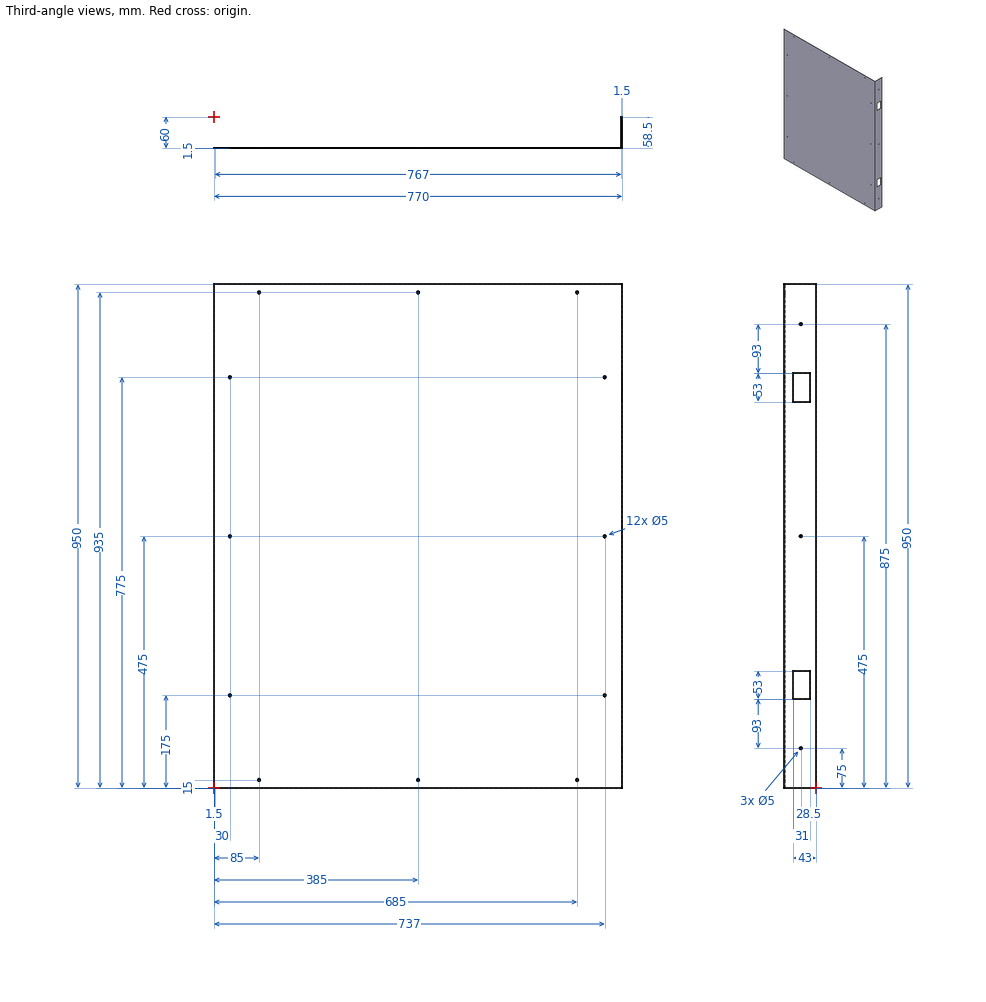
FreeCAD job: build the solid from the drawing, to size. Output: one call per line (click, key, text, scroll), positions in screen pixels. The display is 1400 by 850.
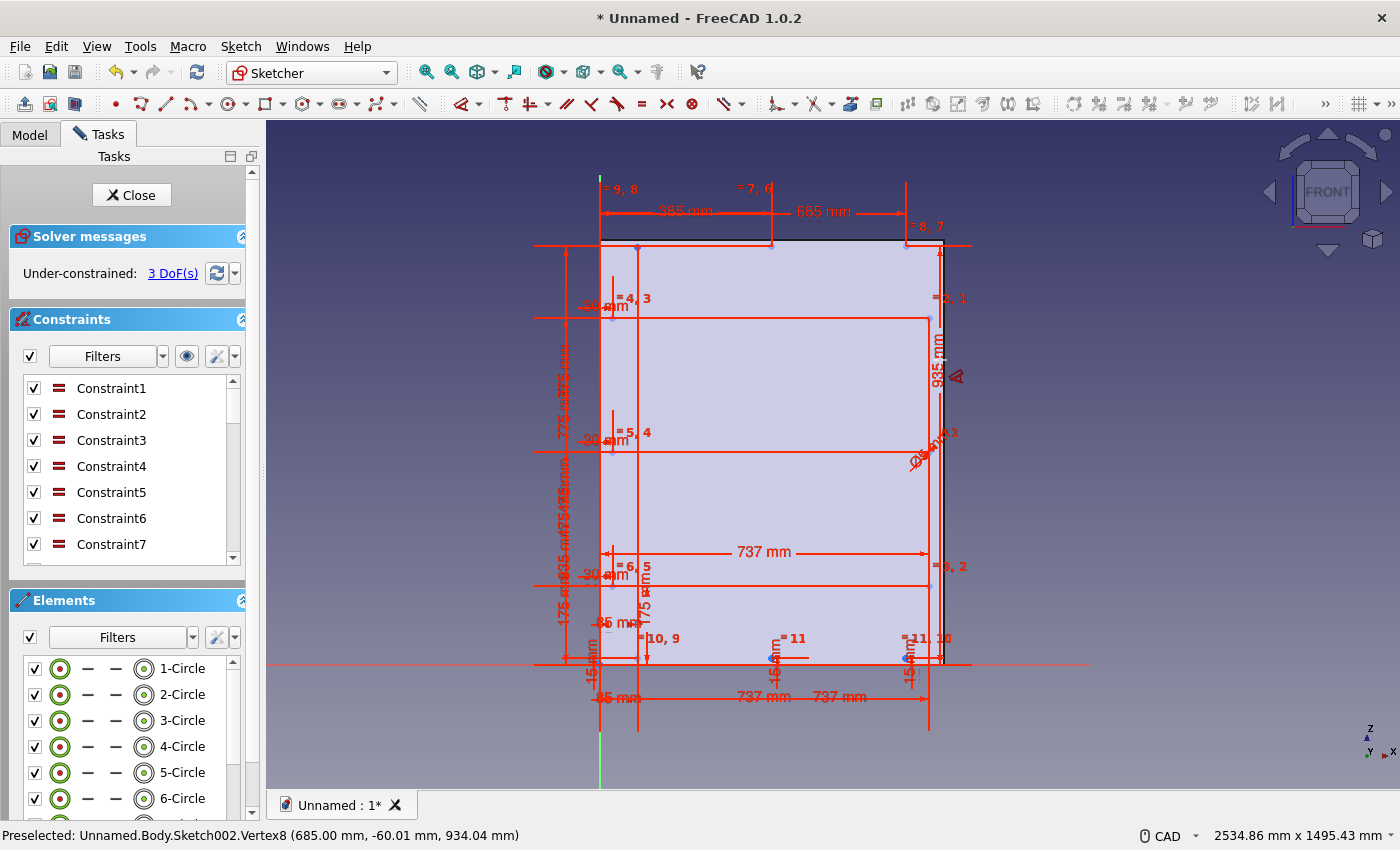
click(638, 247)
click(672, 360)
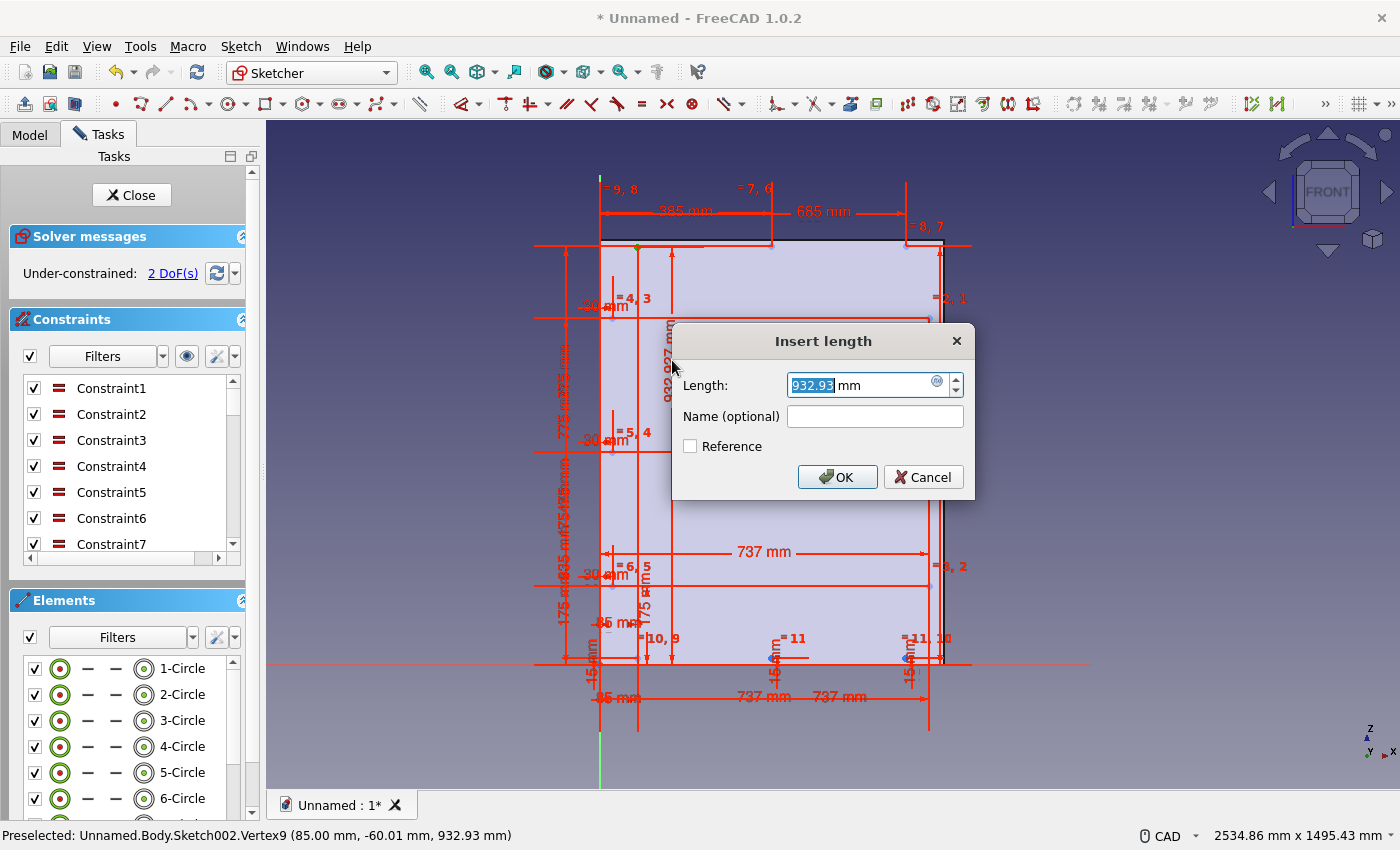
text(935)
key(Return)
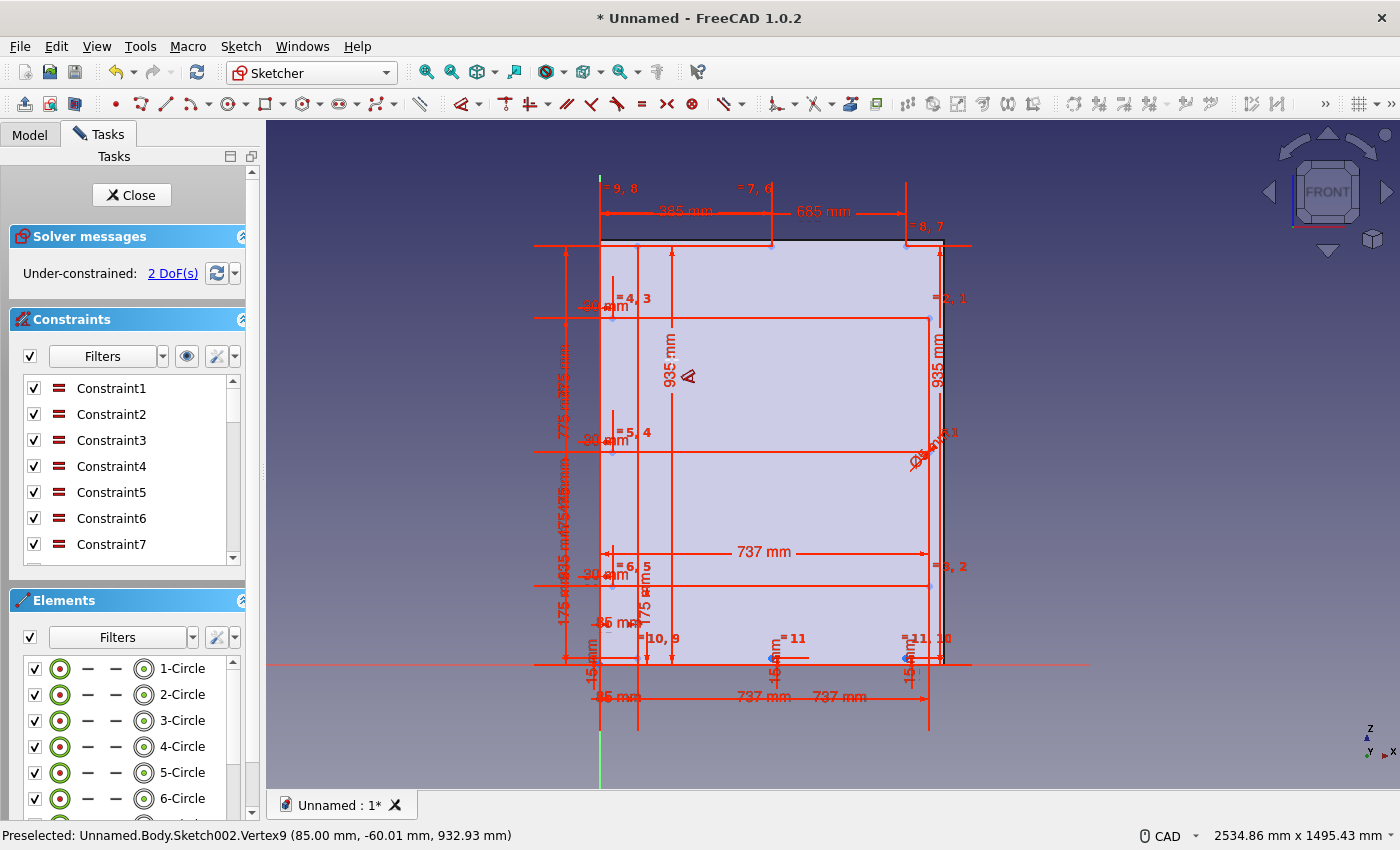
click(906, 658)
click(753, 624)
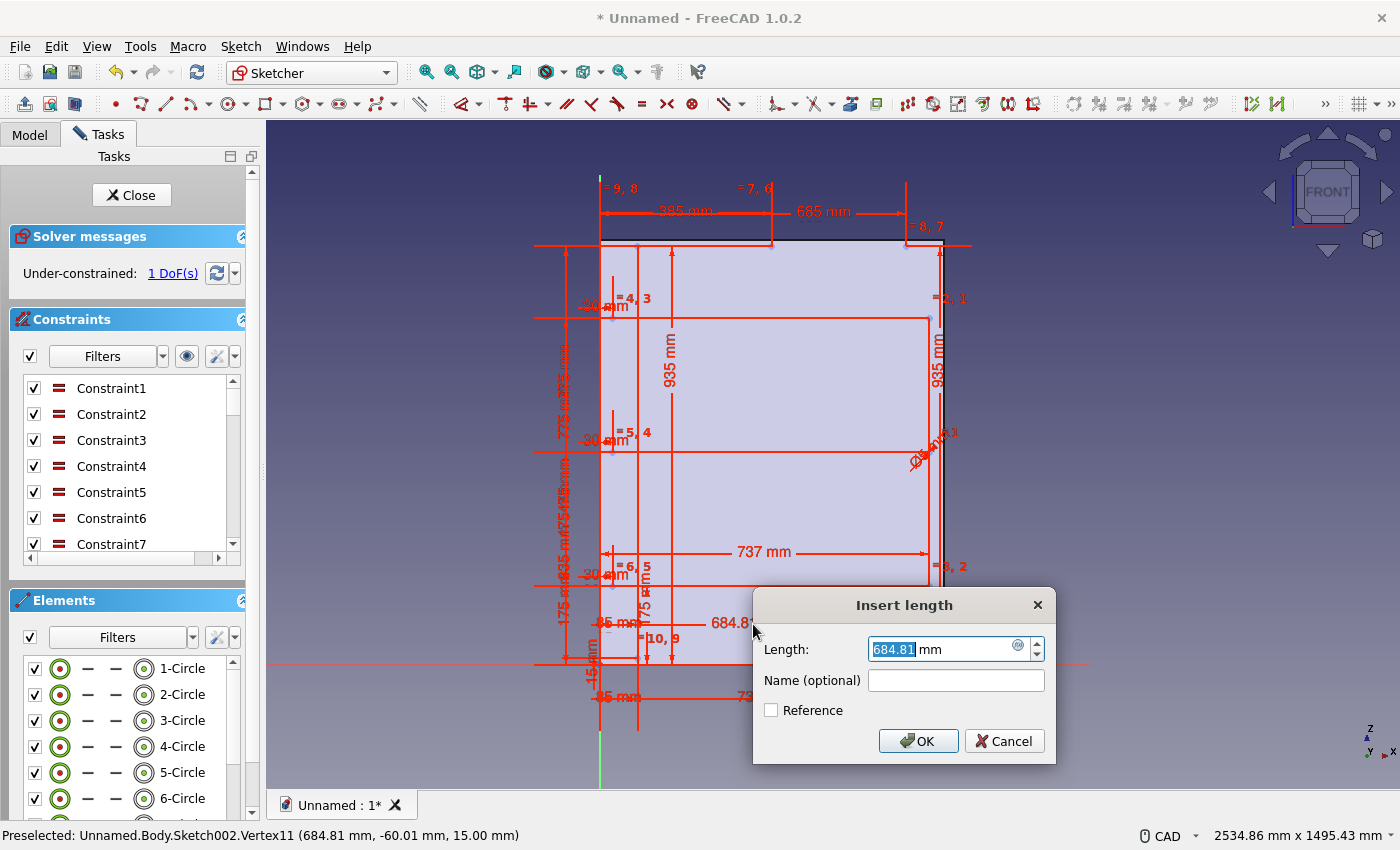
text(685)
key(Return)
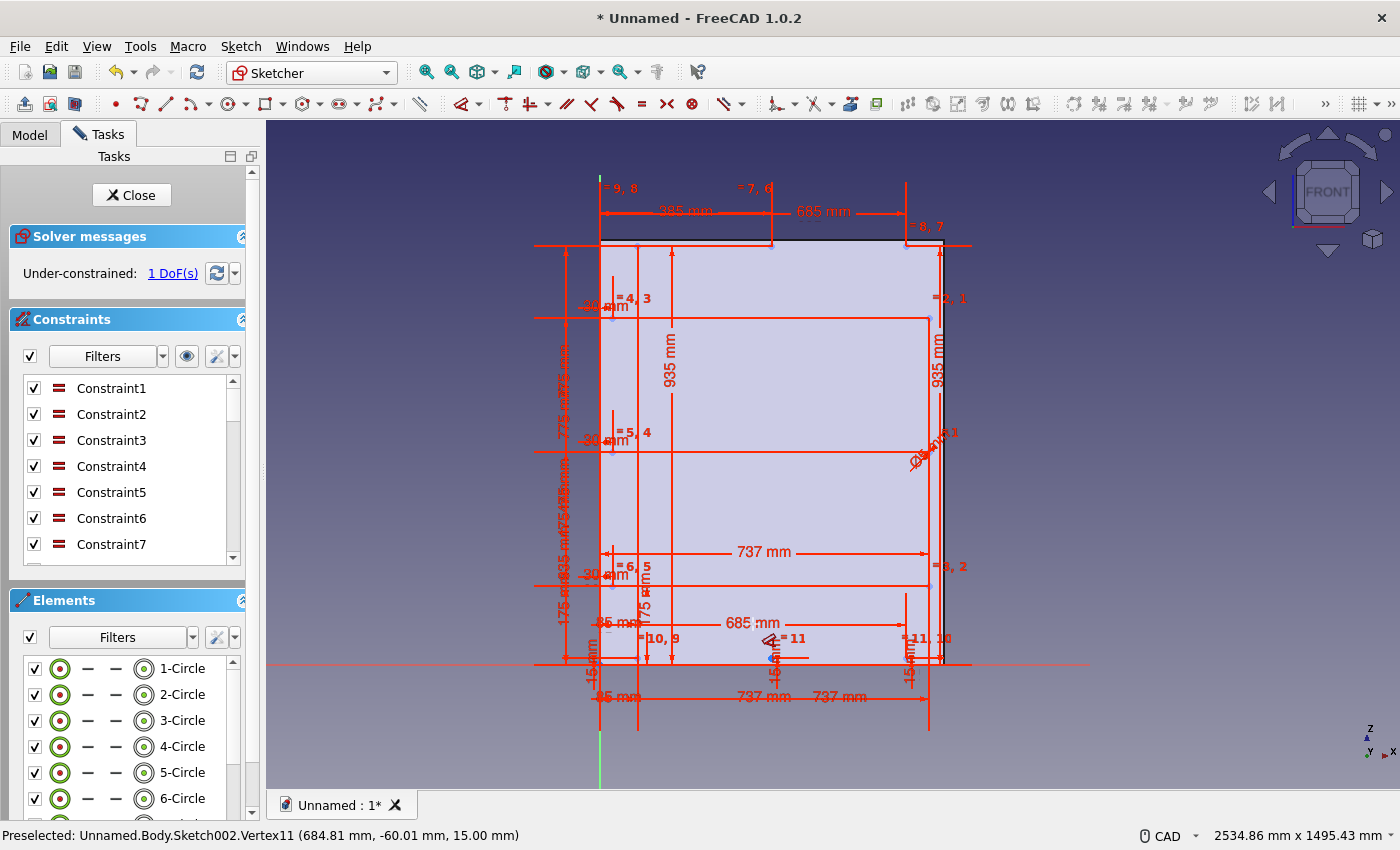
click(772, 658)
click(686, 723)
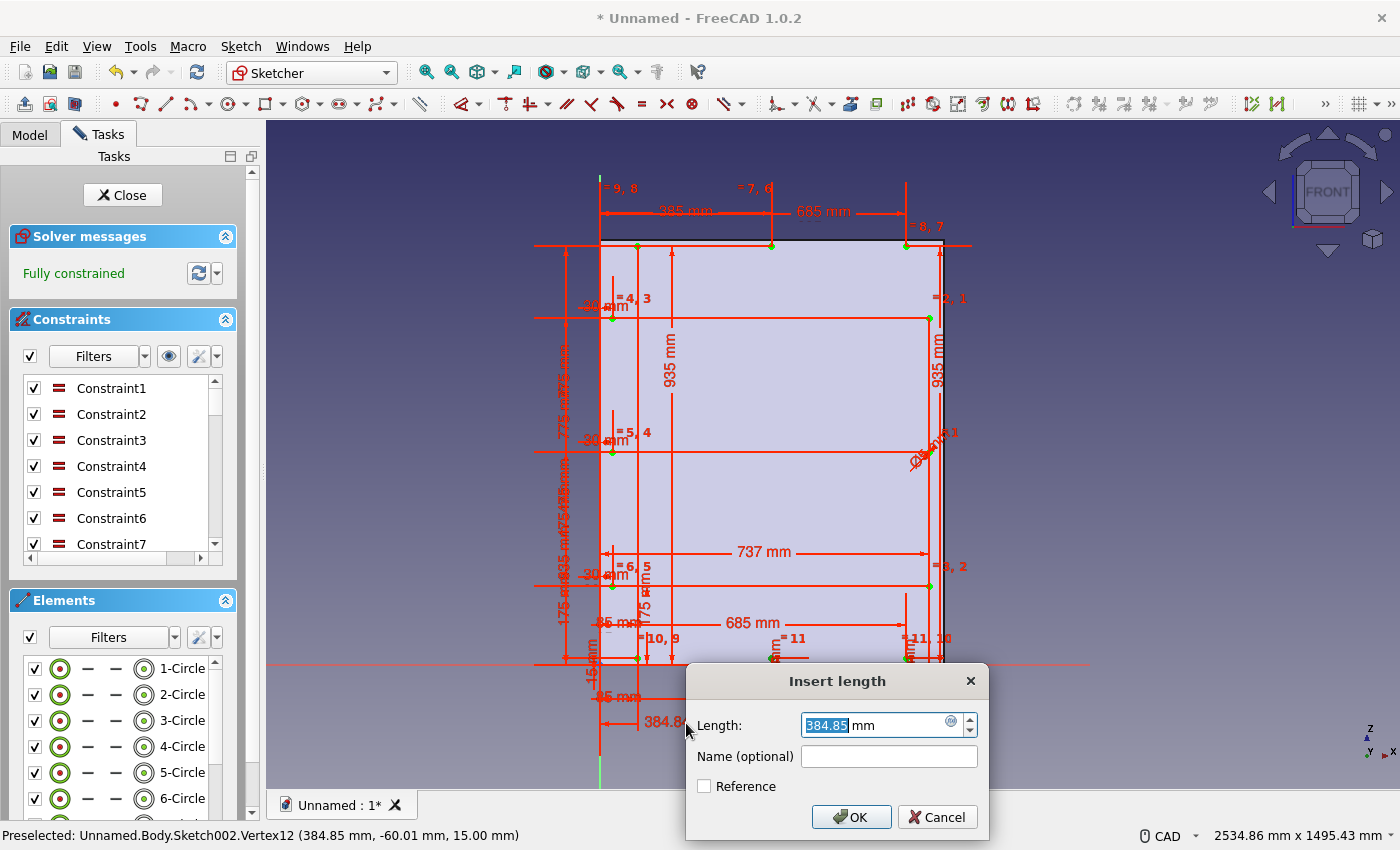
text(385)
key(Return)
key(Escape)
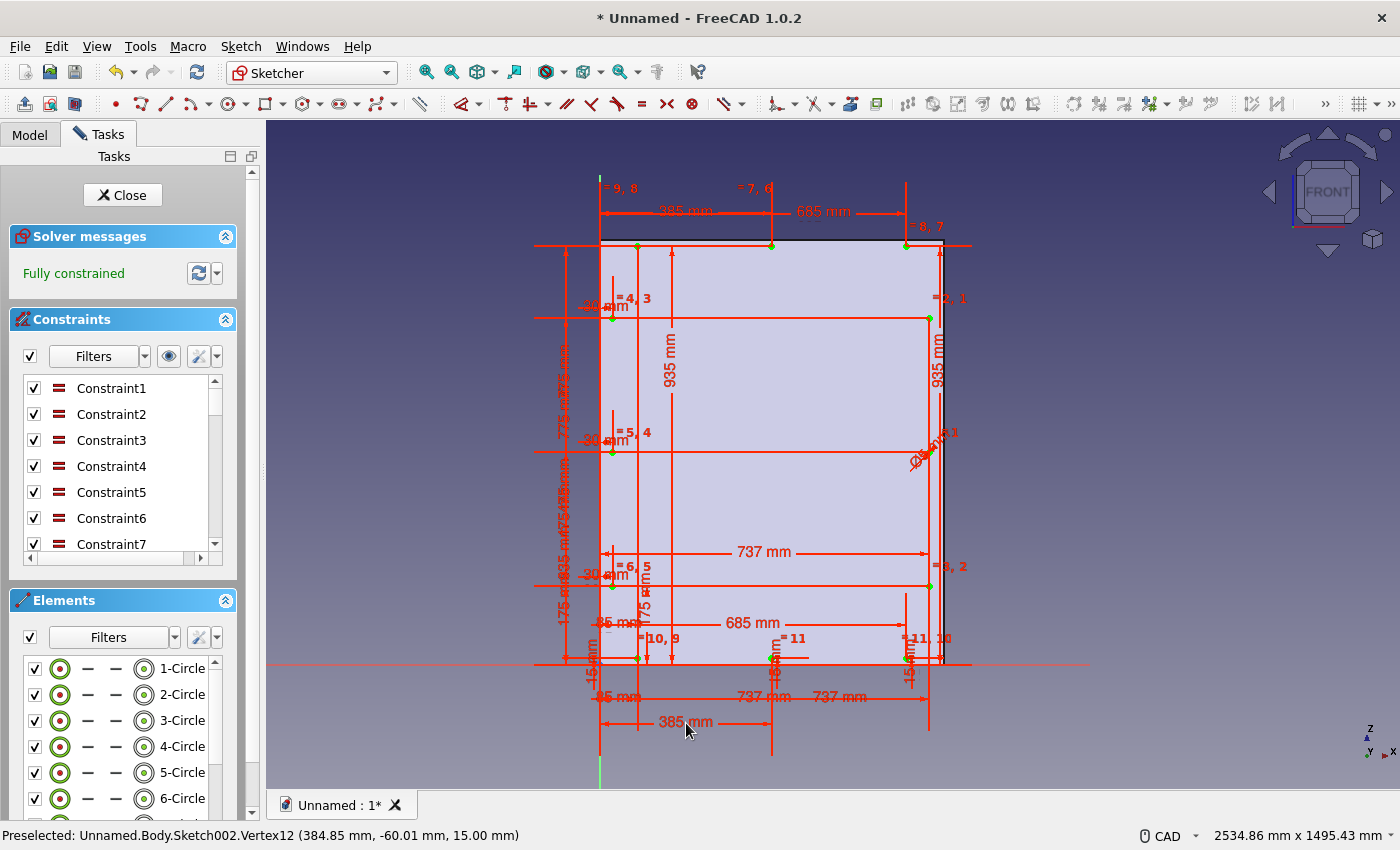
click(123, 195)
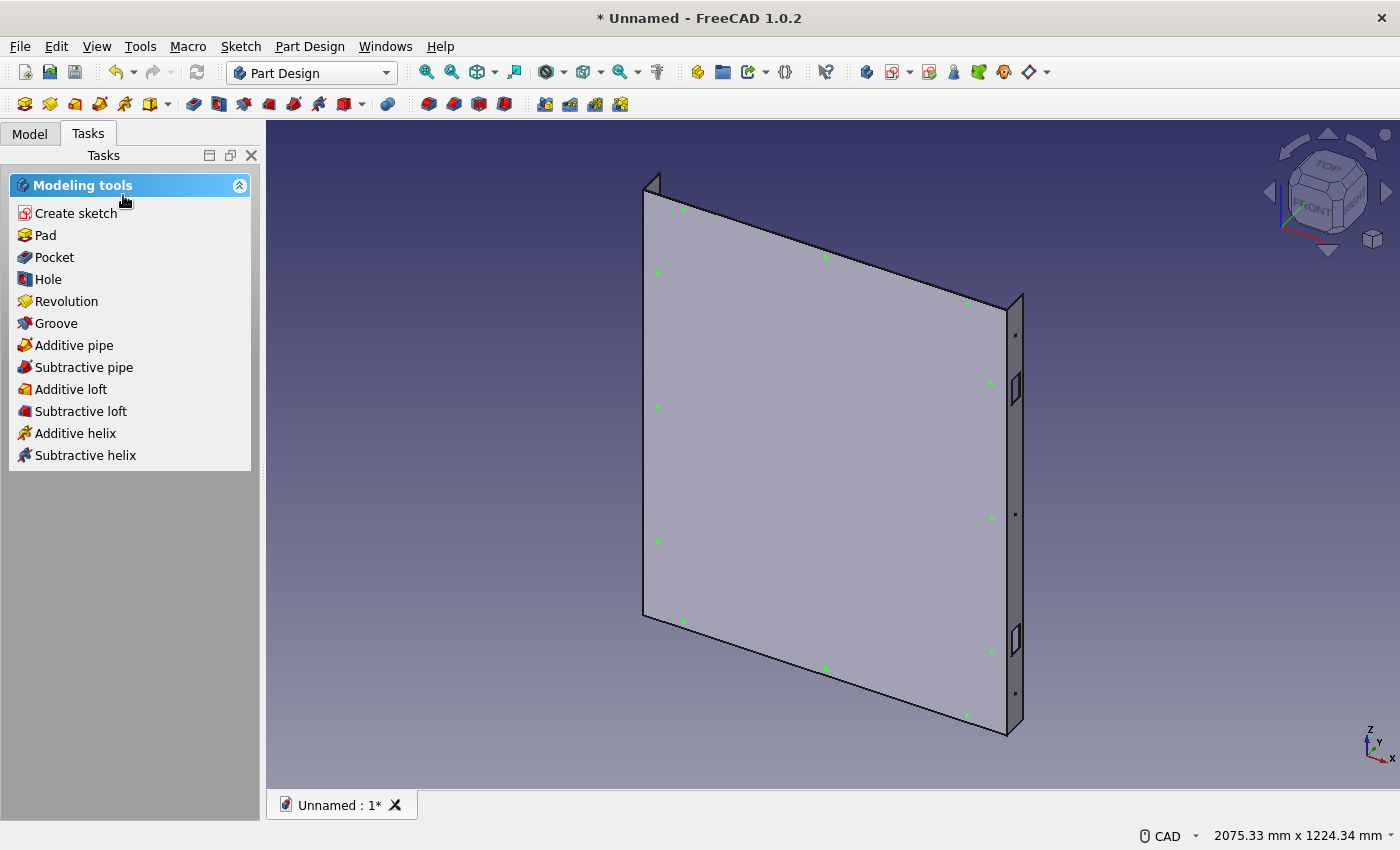
click(194, 104)